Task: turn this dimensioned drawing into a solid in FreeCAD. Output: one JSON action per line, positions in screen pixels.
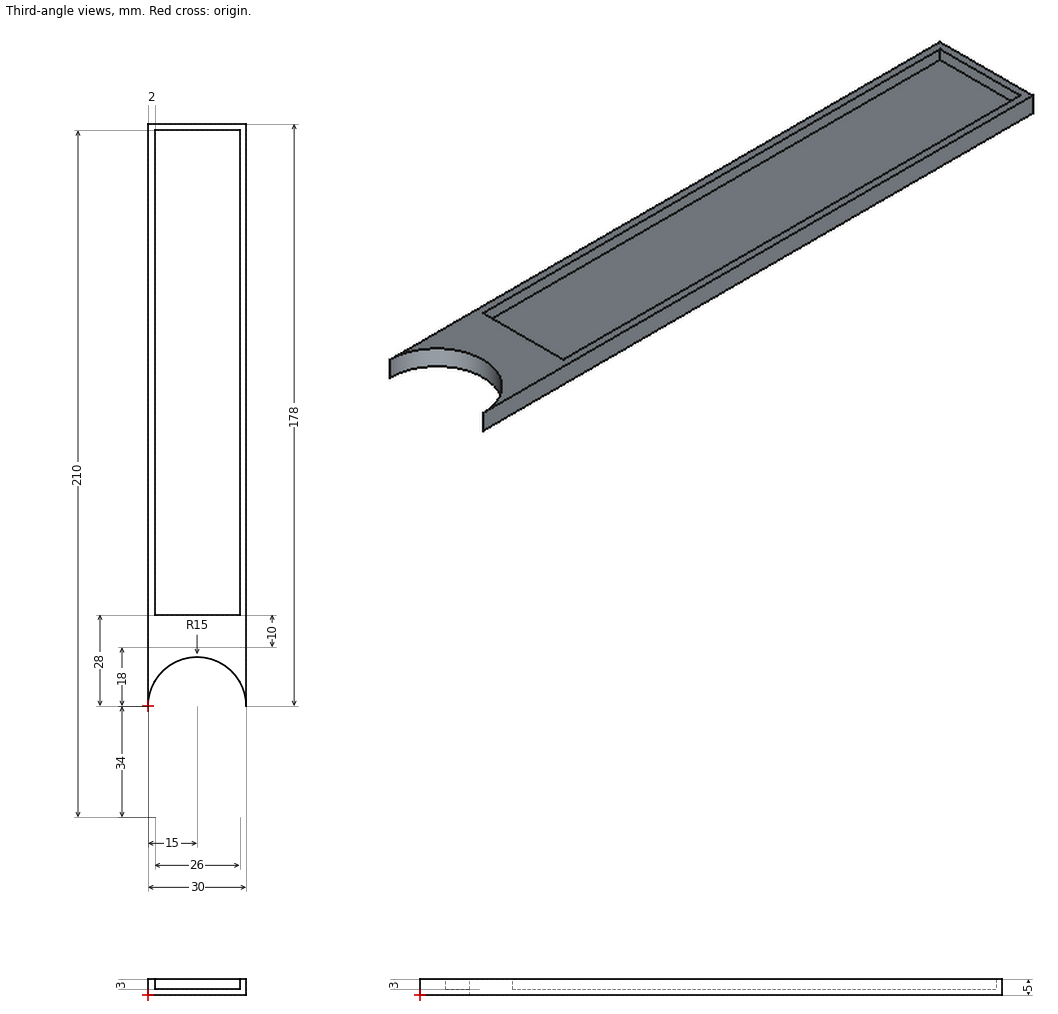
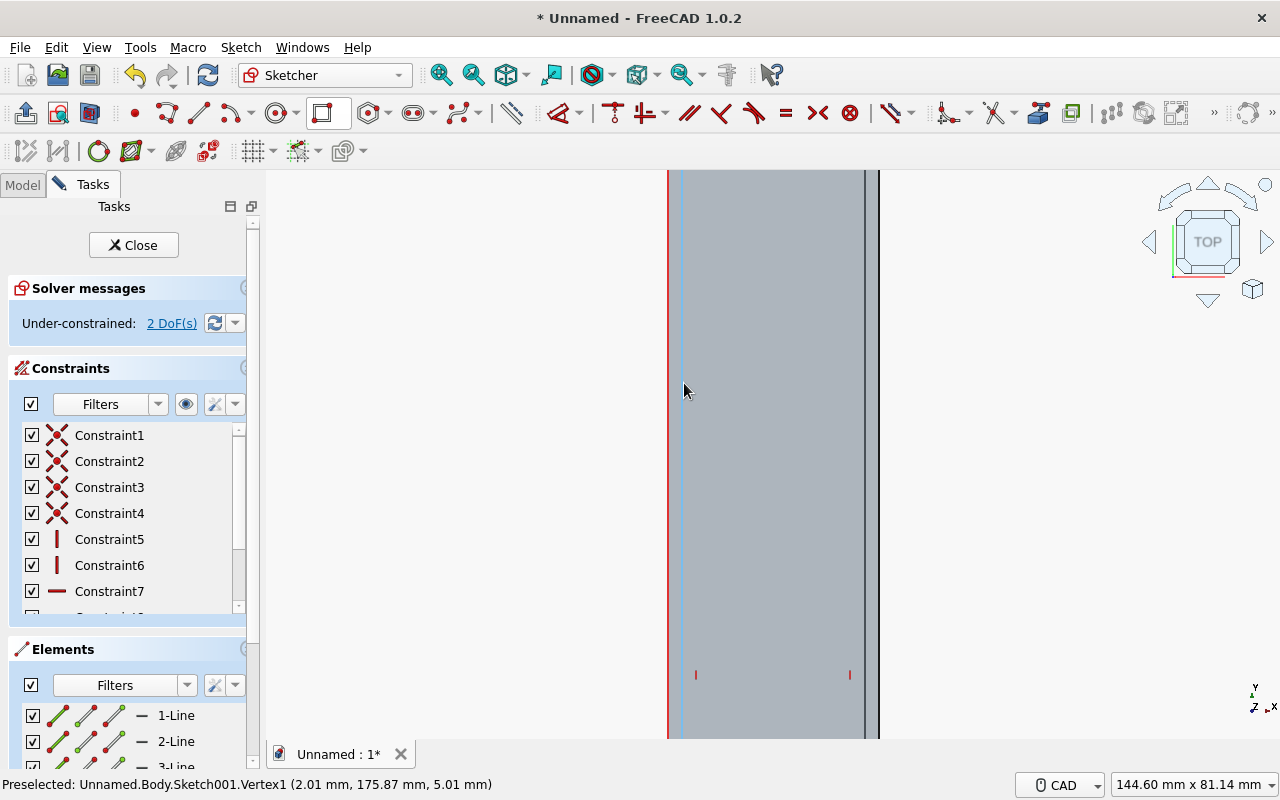
{"action": "left_click", "coordinate": [682, 380]}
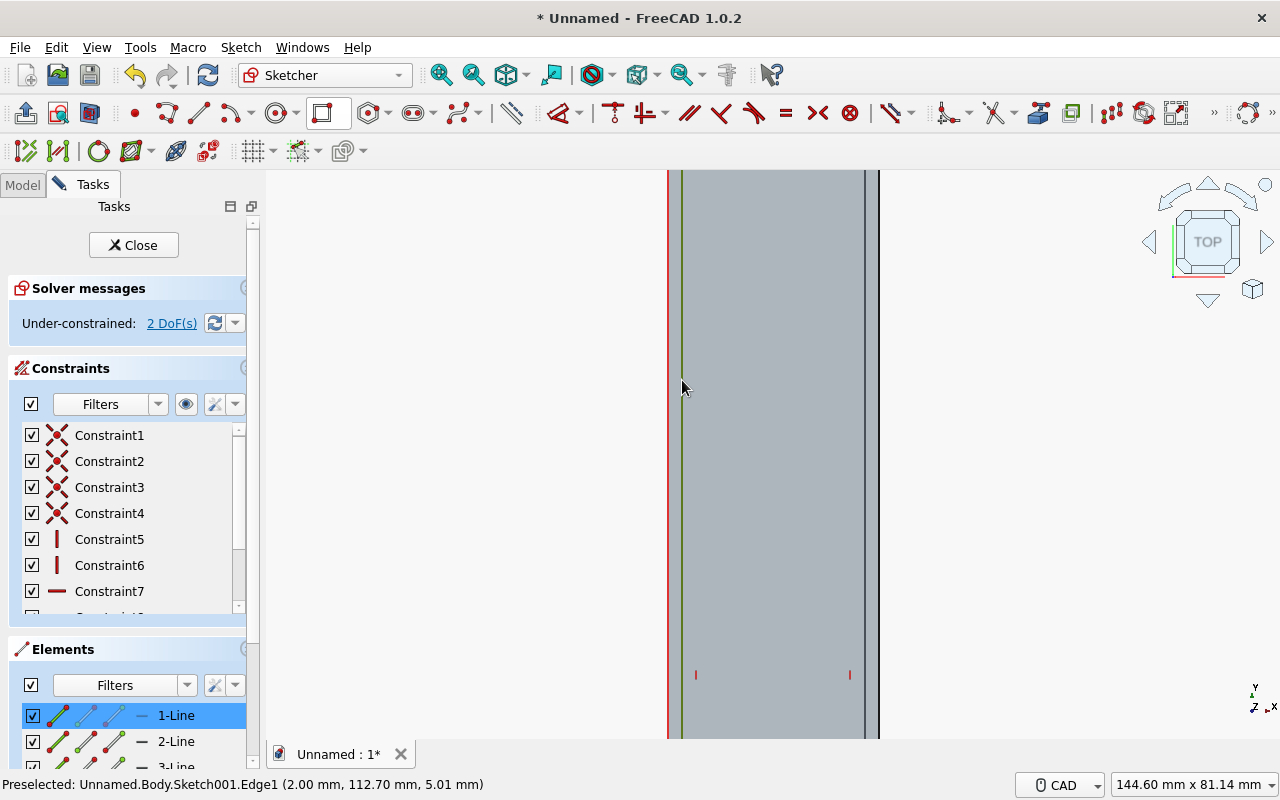
{"action": "key", "text": "i"}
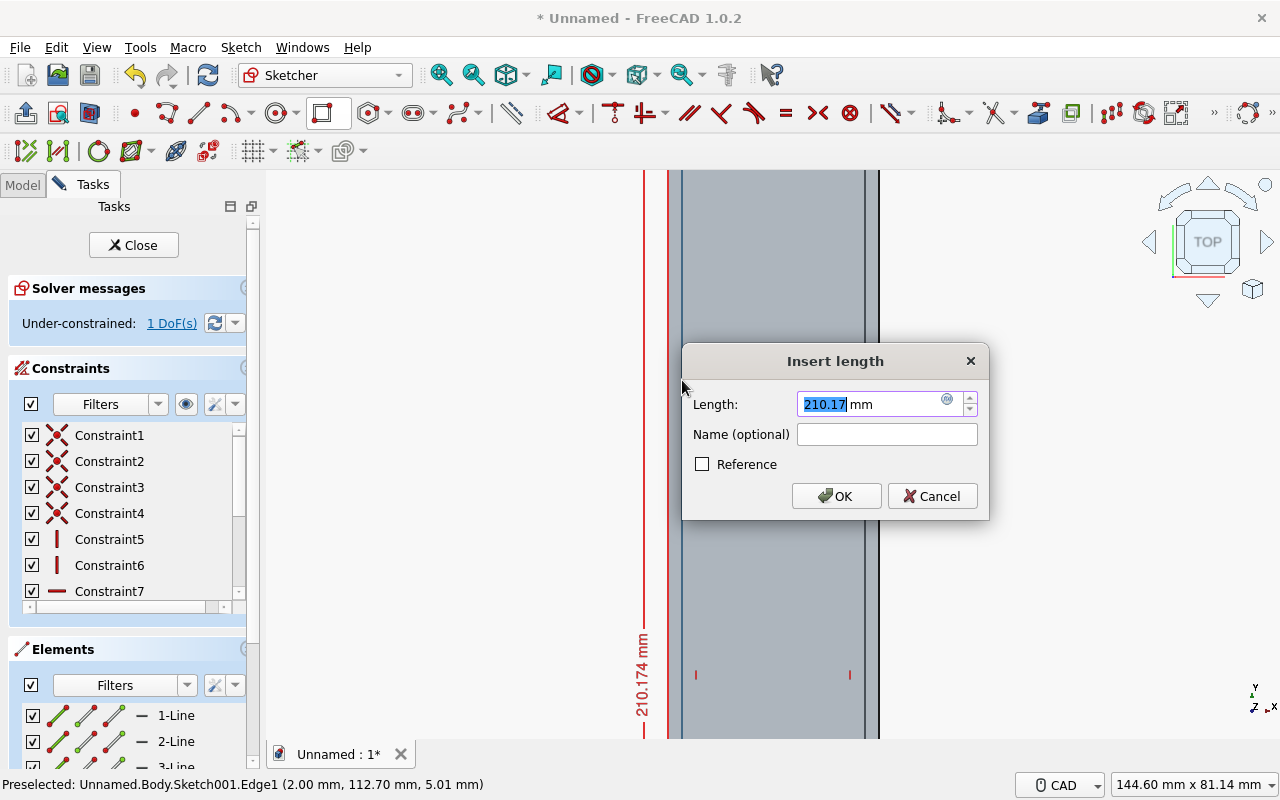
{"action": "type", "text": "210"}
{"action": "key", "text": "Return"}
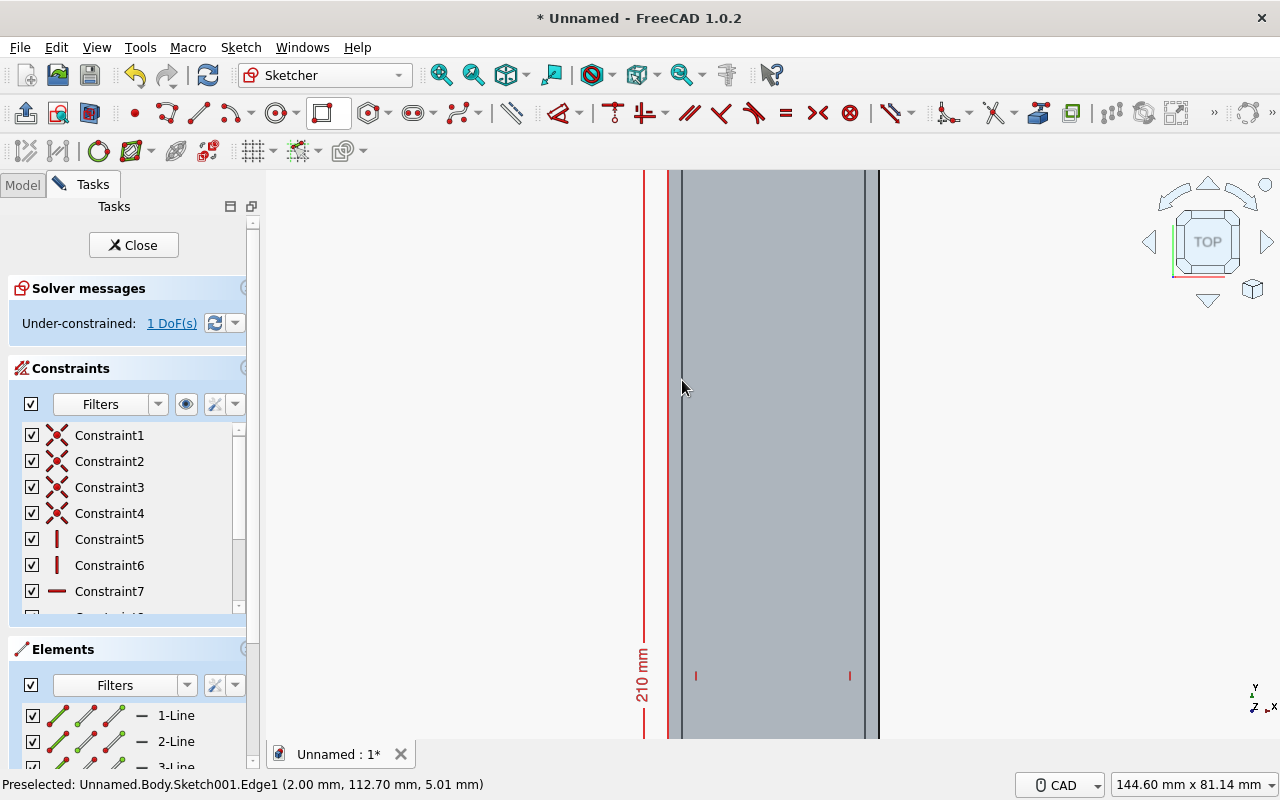
{"action": "scroll", "coordinate": [684, 383], "scroll_direction": "down", "scroll_amount": 7}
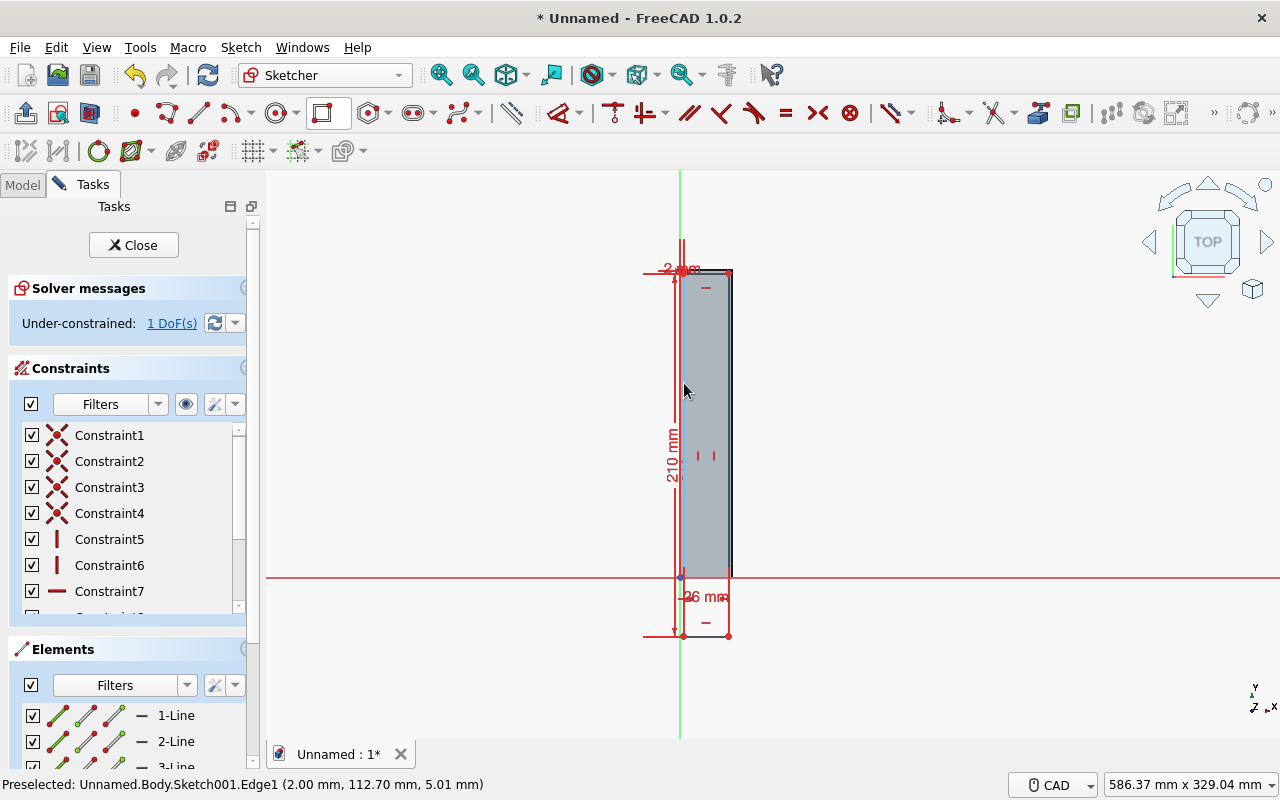
{"action": "left_click", "coordinate": [684, 637]}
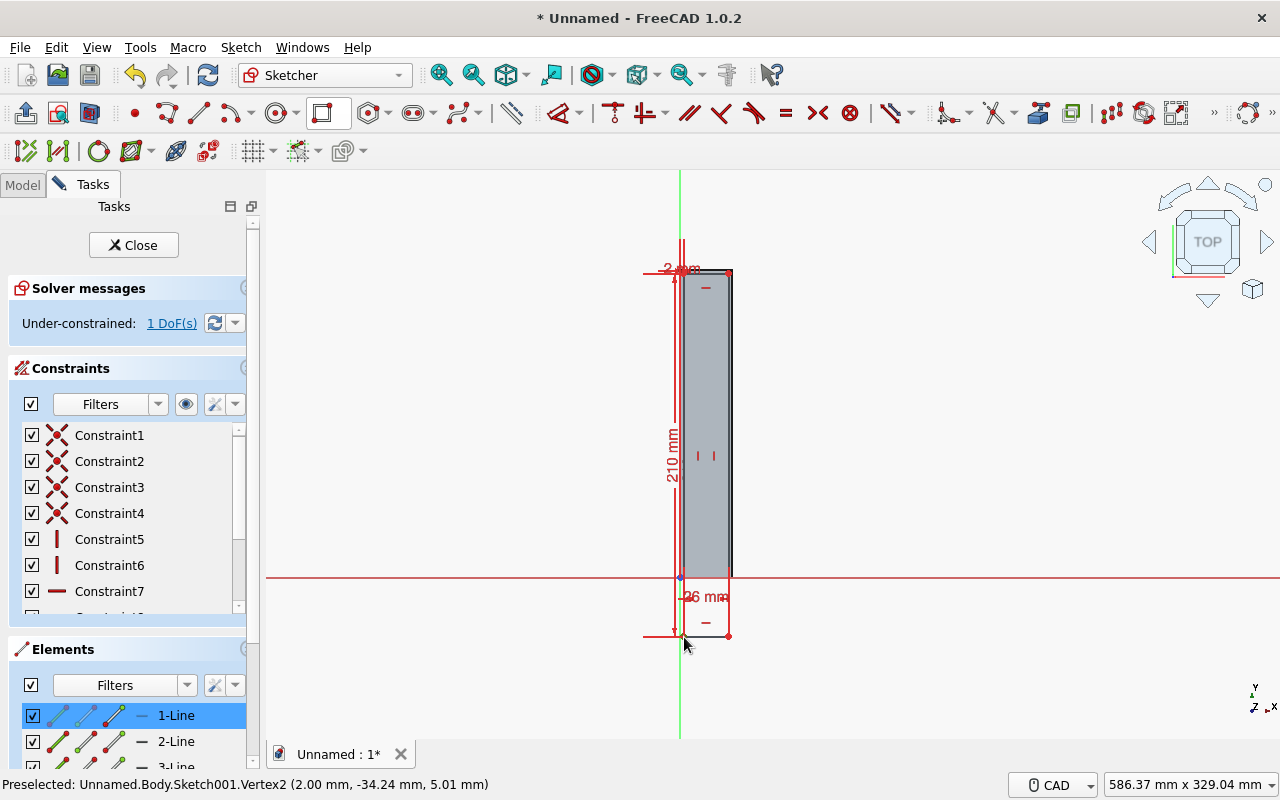
{"action": "key", "text": "i"}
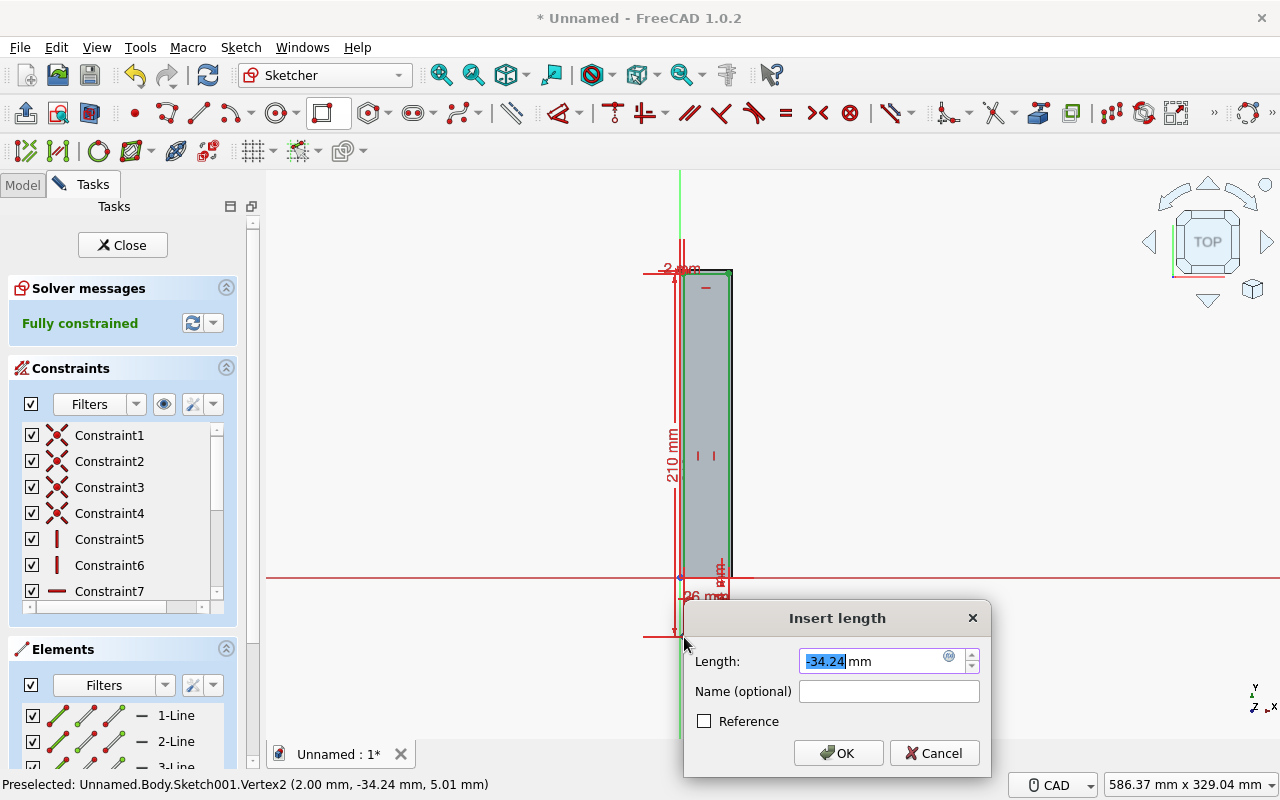
{"action": "type", "text": "-34"}
{"action": "key", "text": "Return"}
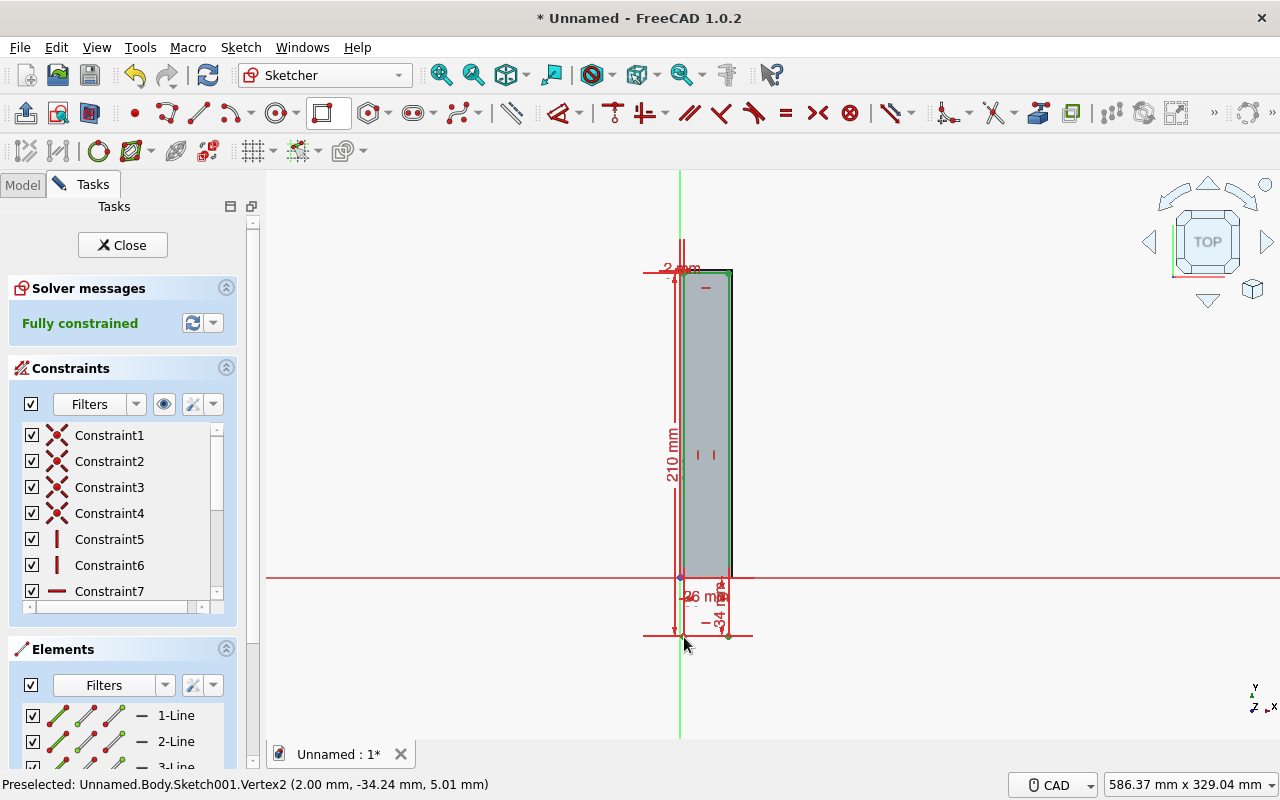
{"action": "left_click", "coordinate": [123, 245]}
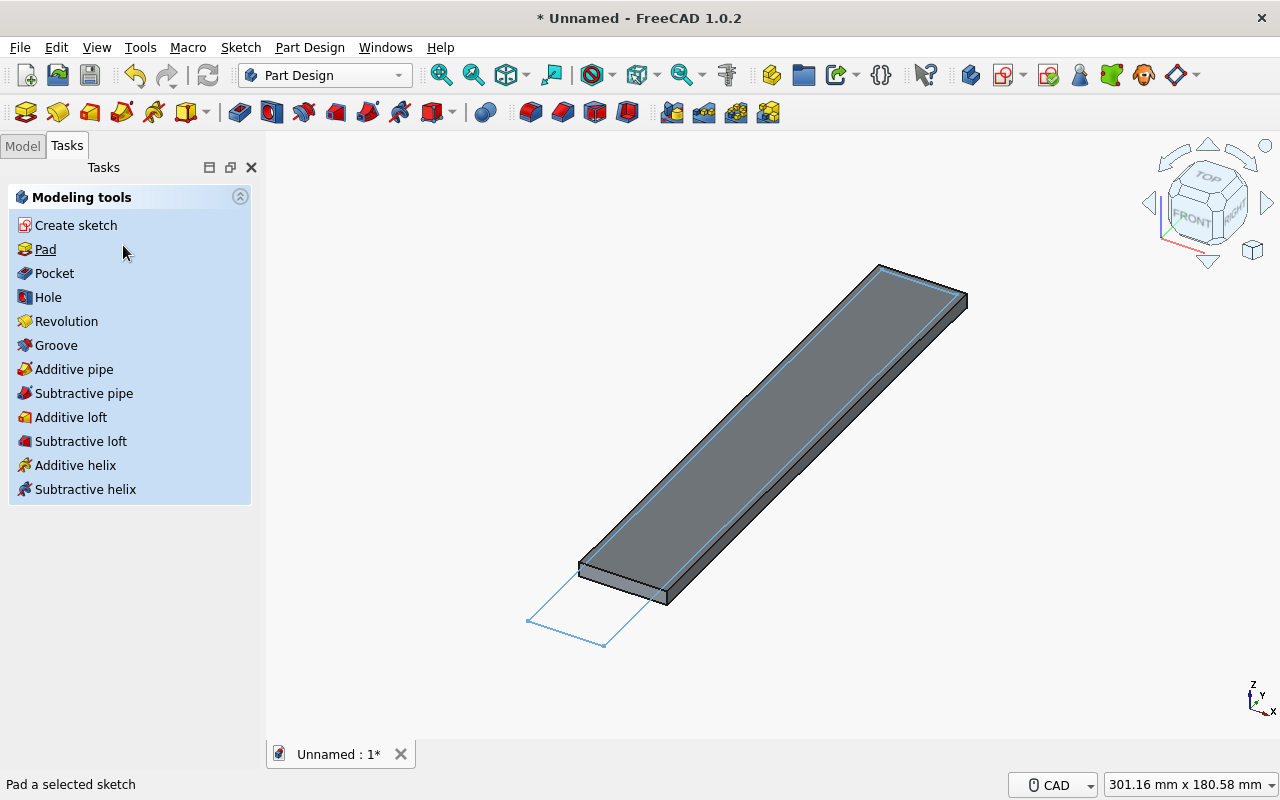
{"action": "left_click", "coordinate": [240, 112]}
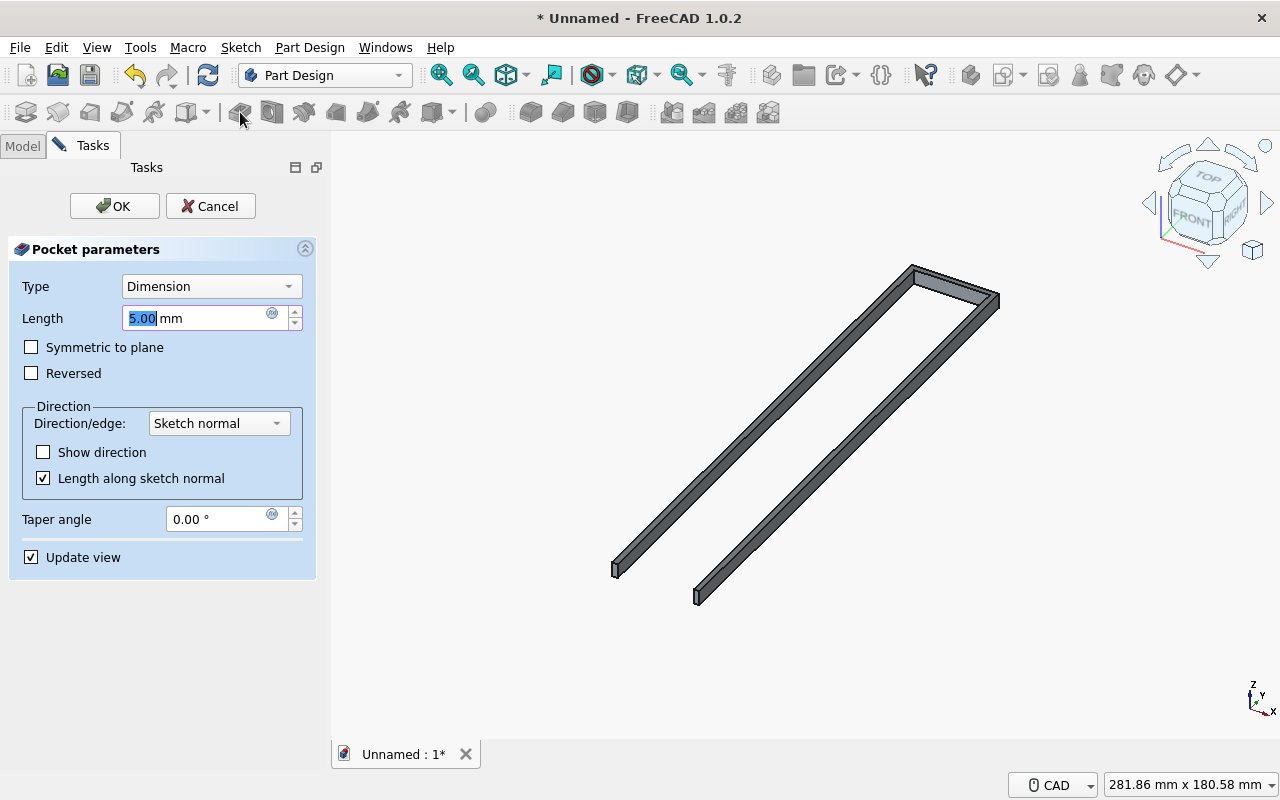
{"action": "type", "text": "3"}
{"action": "key", "text": "Tab"}